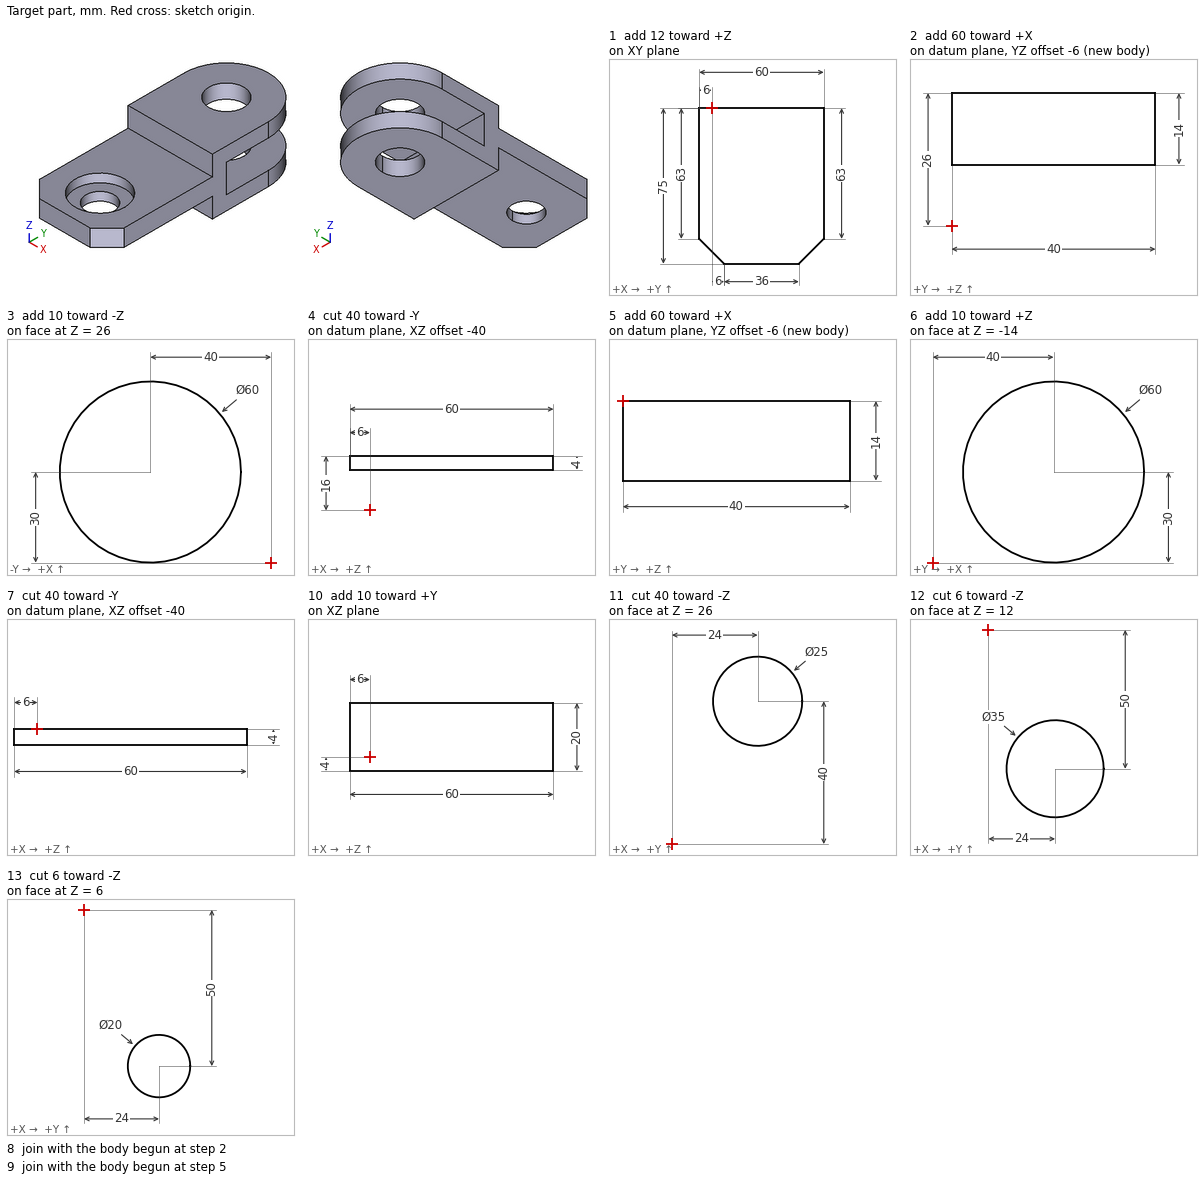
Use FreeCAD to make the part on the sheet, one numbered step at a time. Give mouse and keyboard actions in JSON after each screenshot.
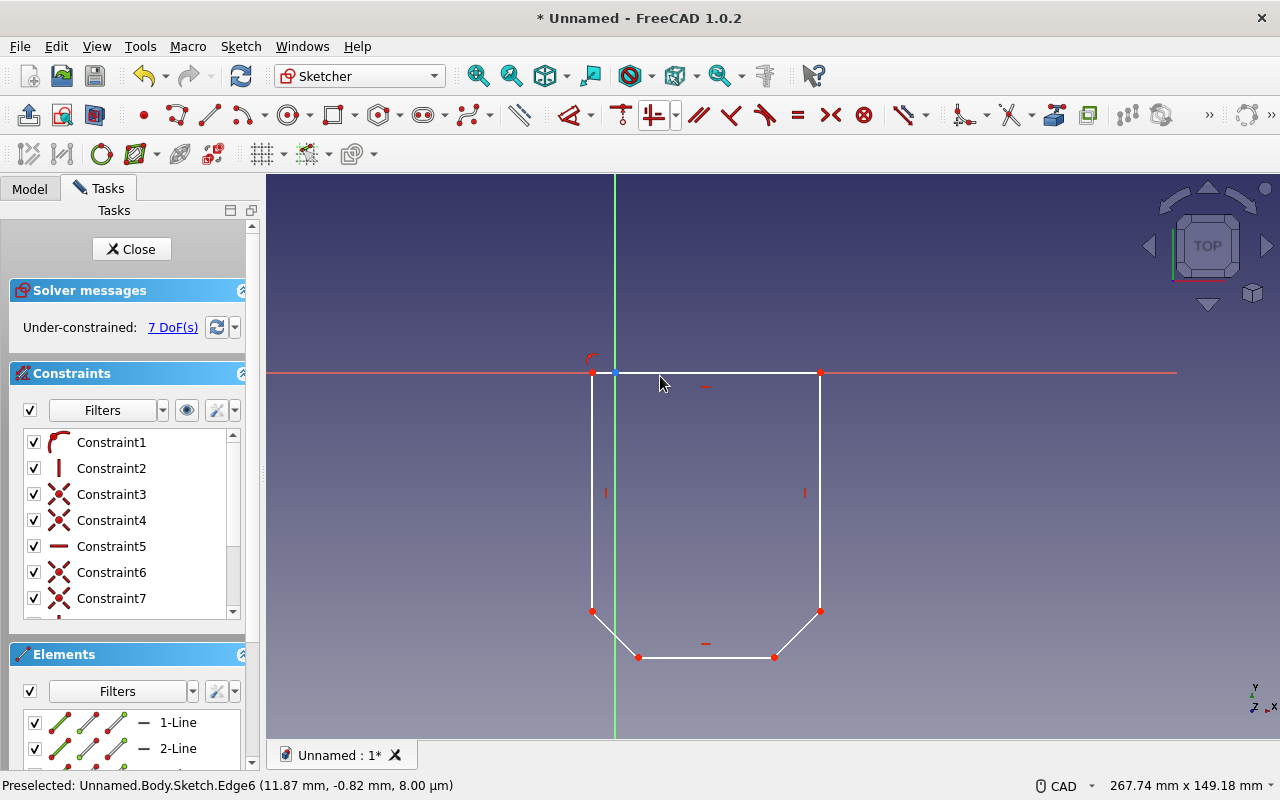
{"action": "left_click", "coordinate": [592, 444]}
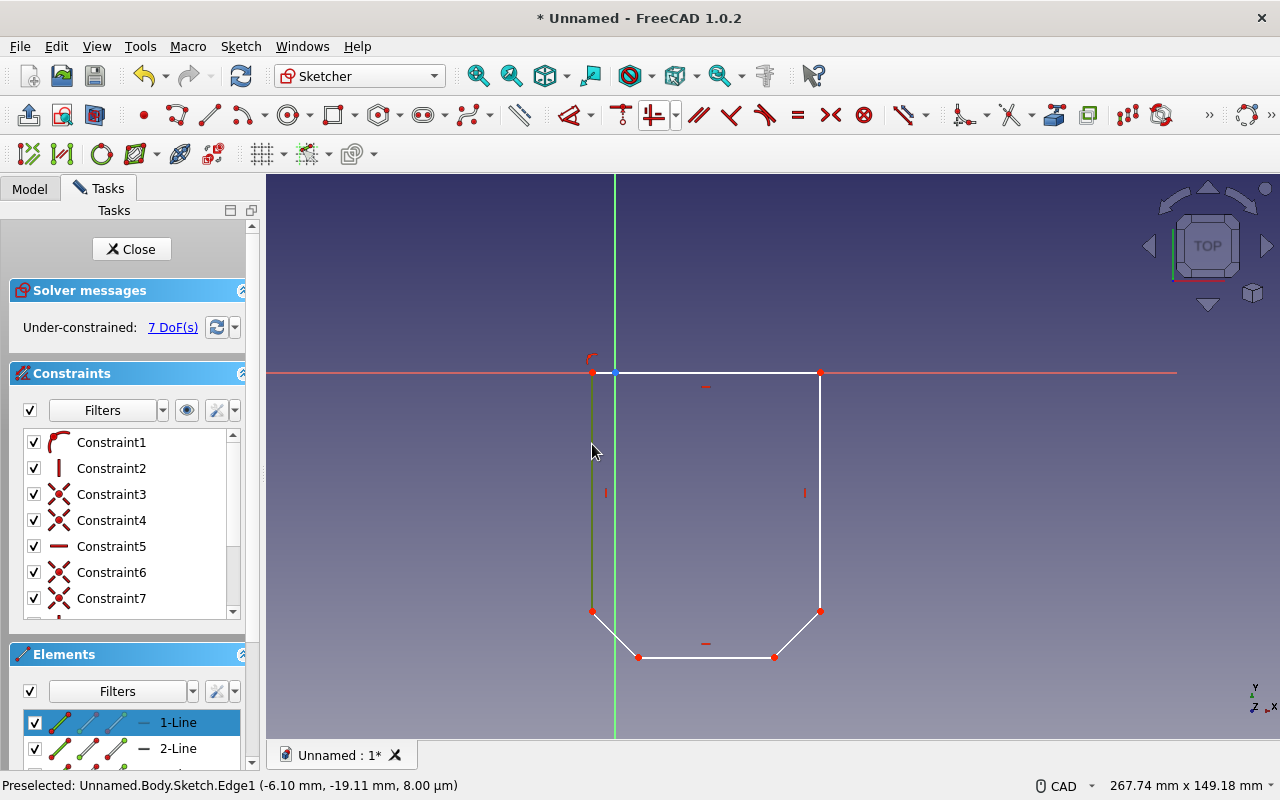
{"action": "left_click", "coordinate": [590, 116]}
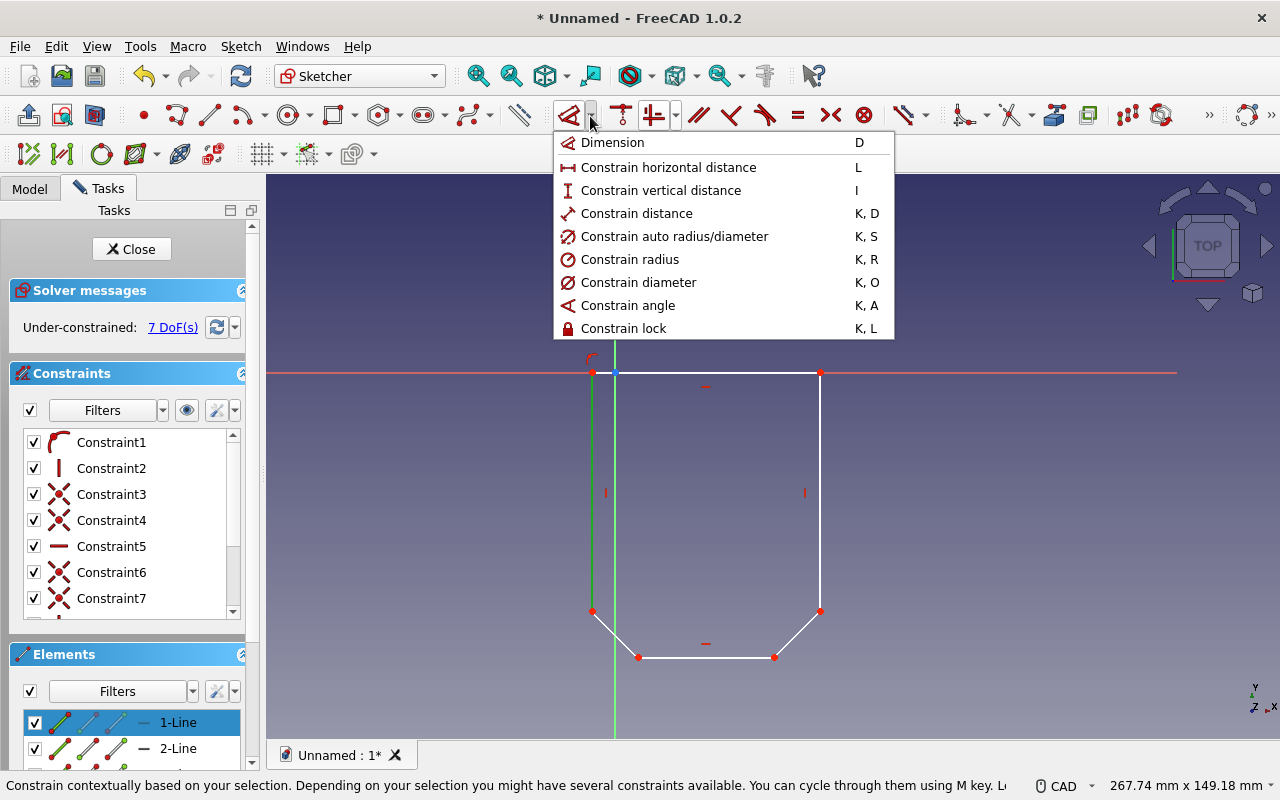
{"action": "left_click", "coordinate": [724, 190]}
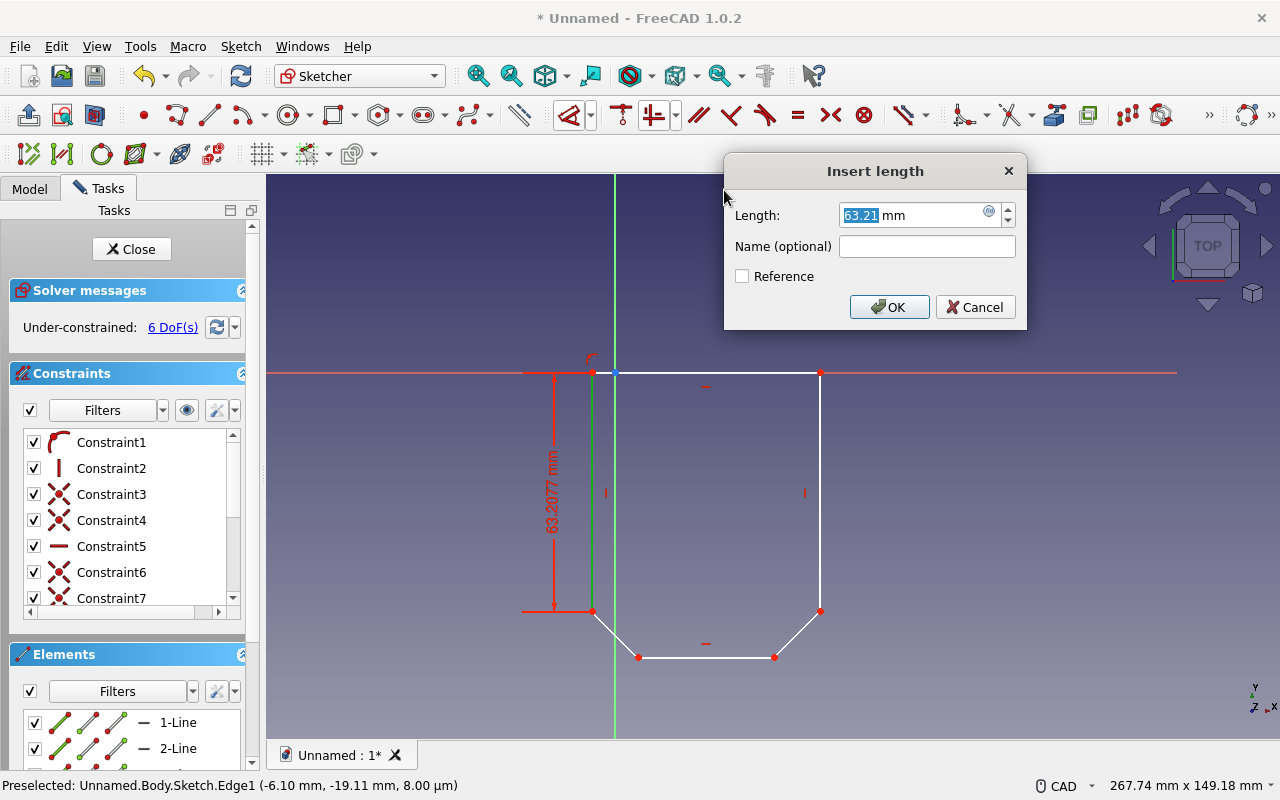
{"action": "type", "text": "63"}
{"action": "key", "text": "Return"}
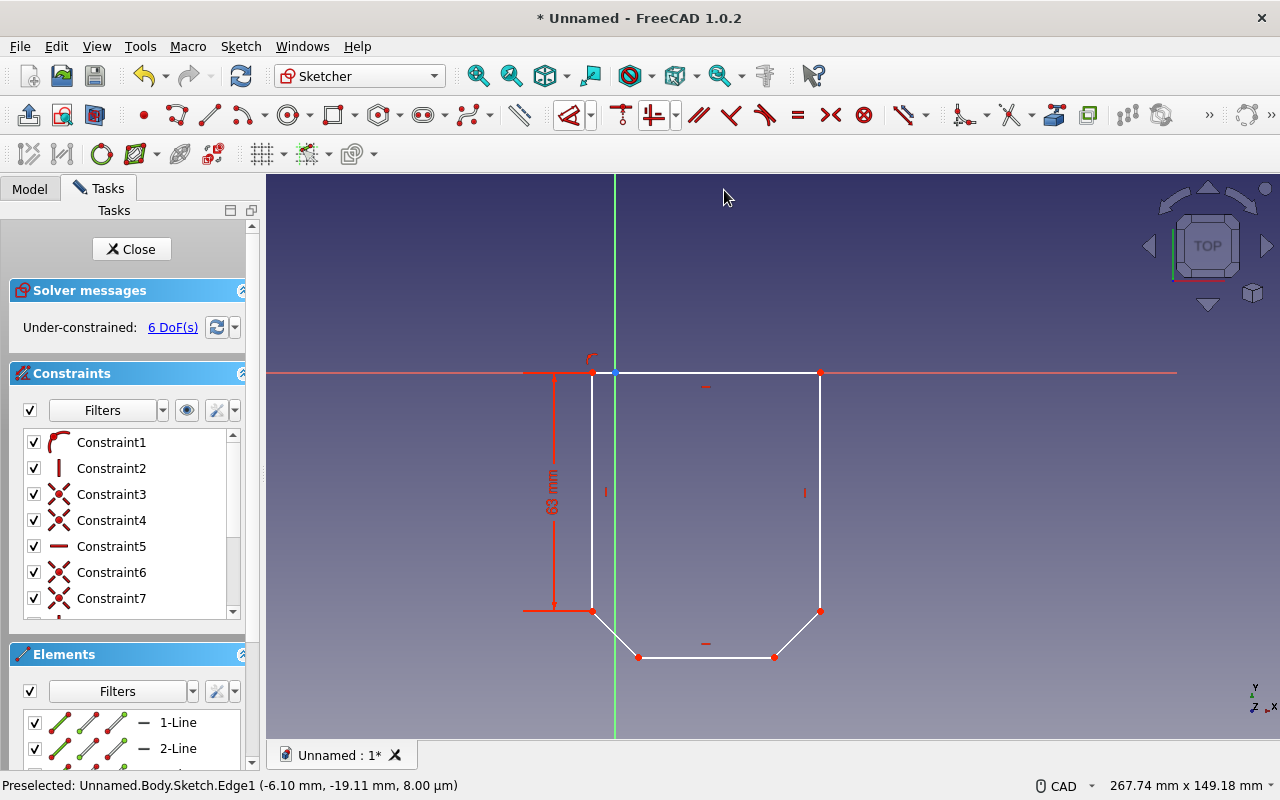
{"action": "left_click", "coordinate": [679, 658]}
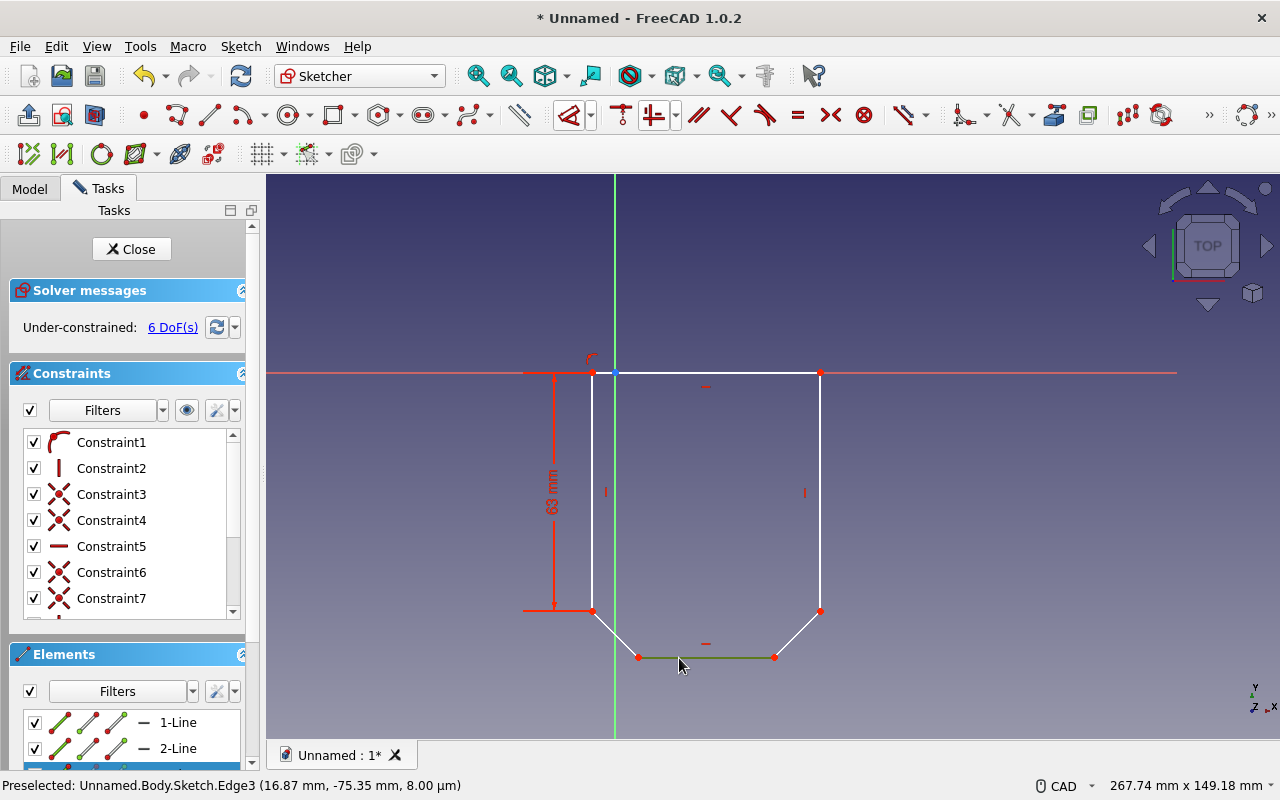
{"action": "left_click", "coordinate": [590, 116]}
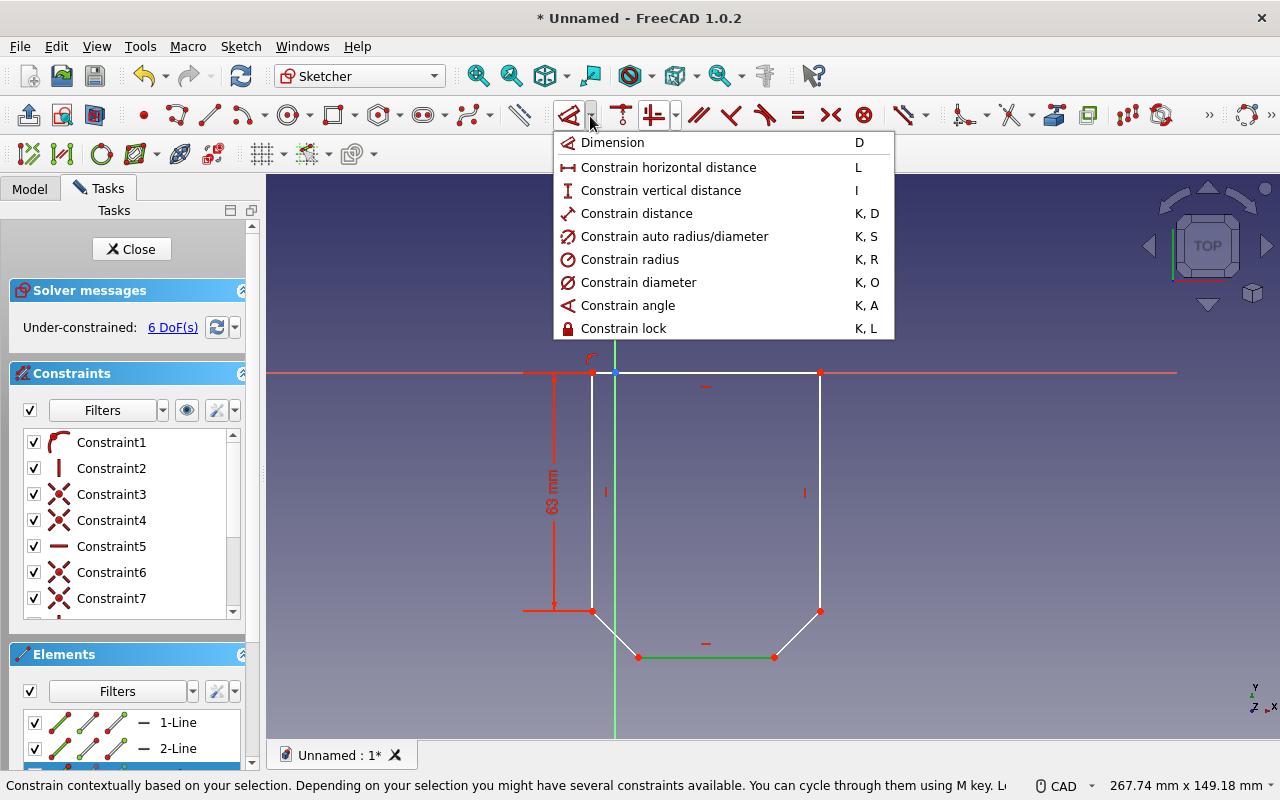
{"action": "left_click", "coordinate": [724, 168]}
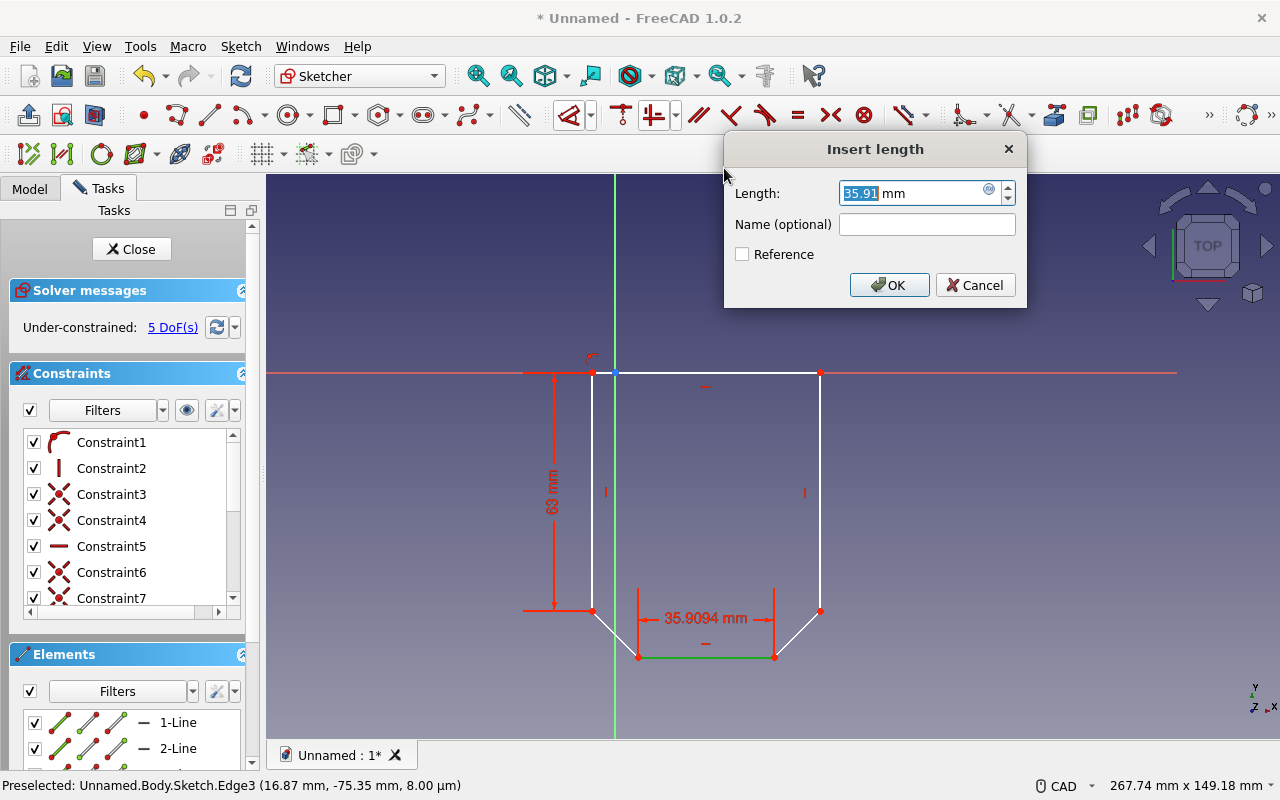
{"action": "type", "text": "36"}
{"action": "key", "text": "Return"}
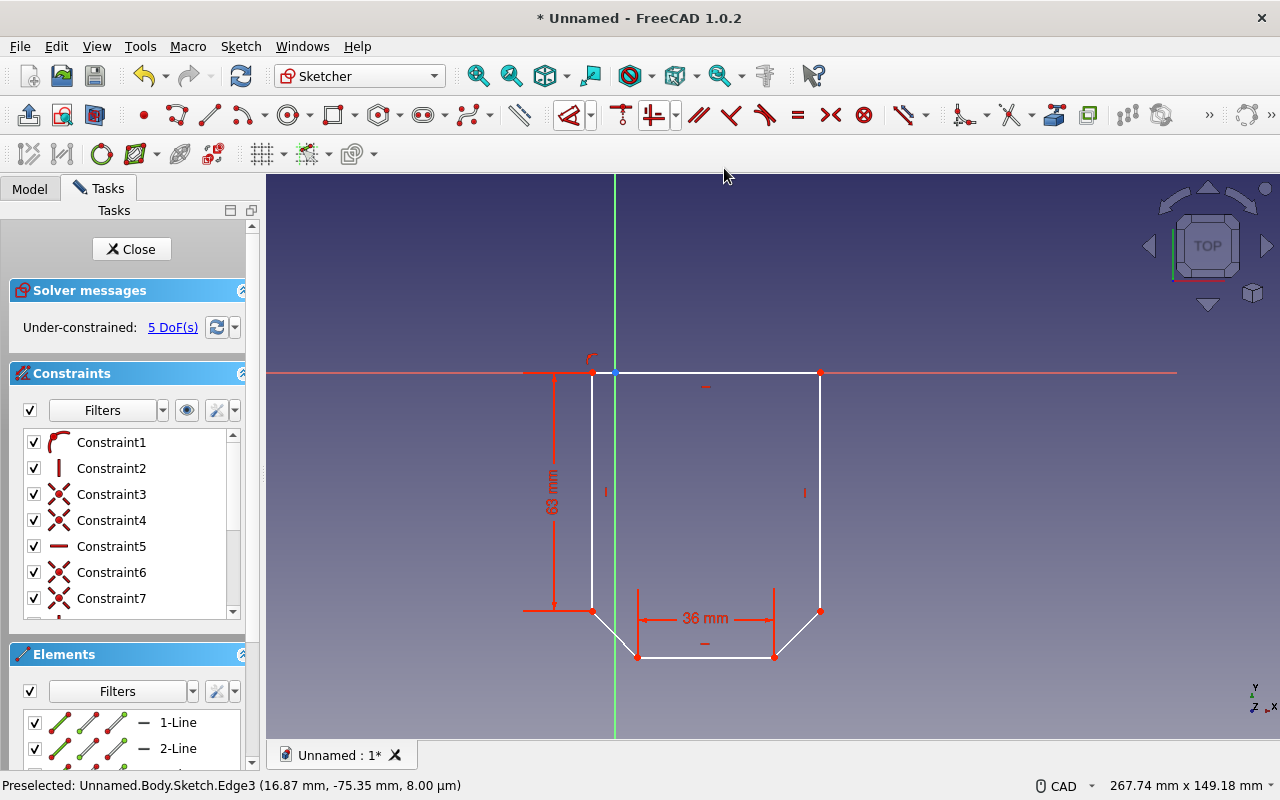
{"action": "left_click", "coordinate": [820, 540]}